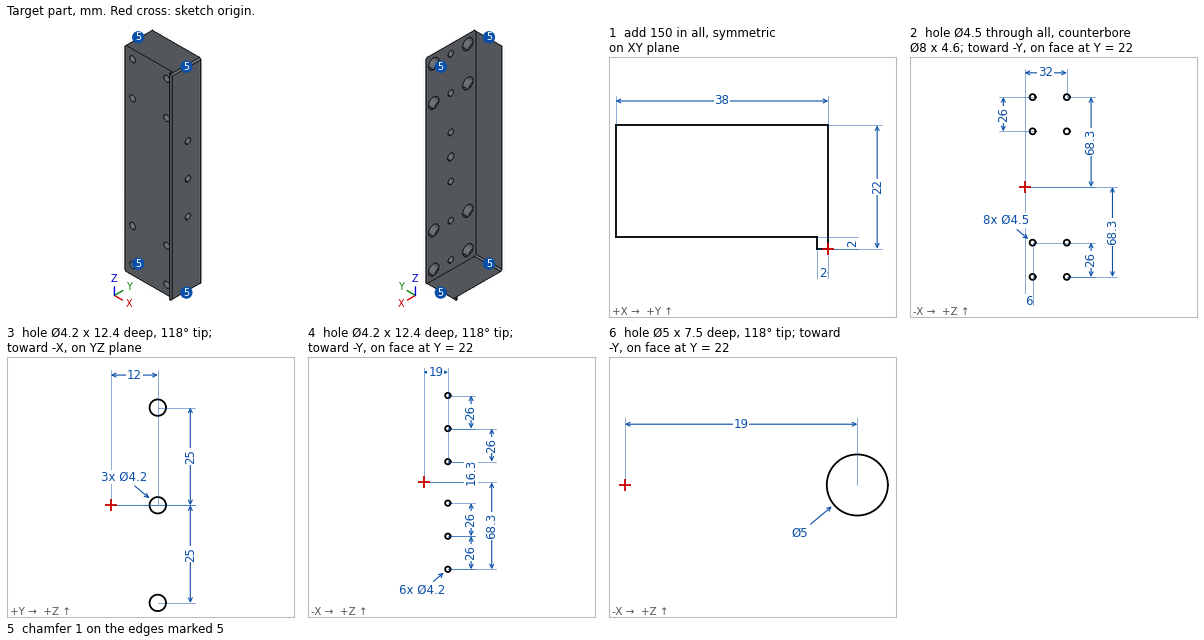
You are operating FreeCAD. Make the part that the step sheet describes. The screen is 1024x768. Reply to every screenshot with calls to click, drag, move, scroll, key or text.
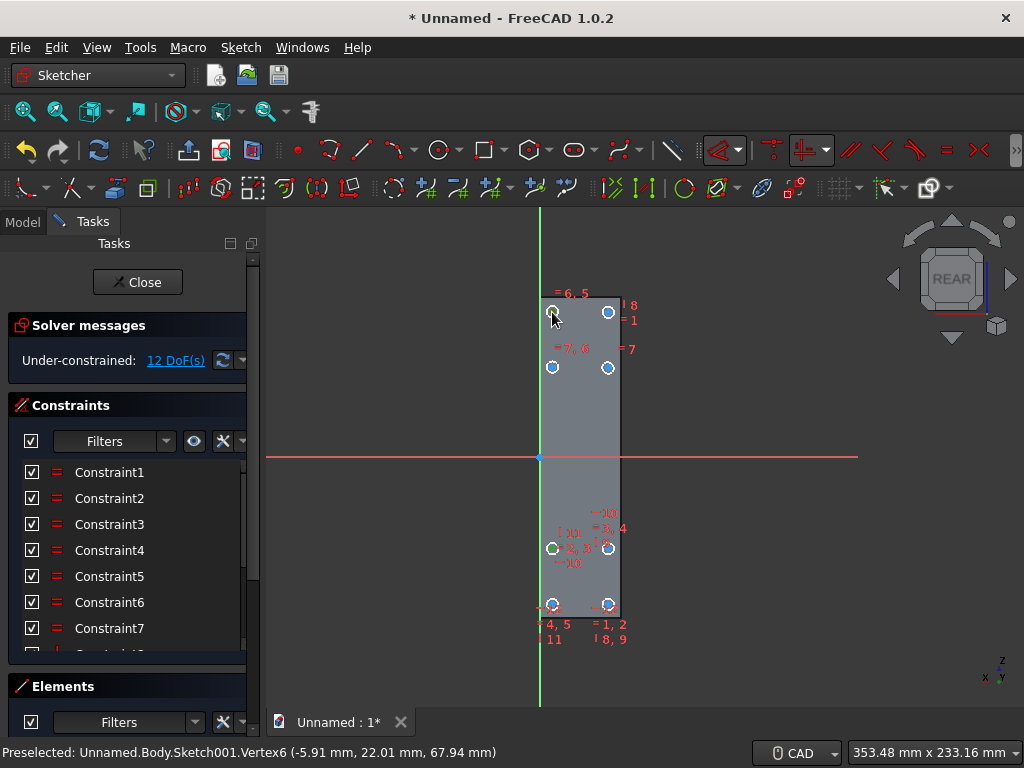
key(v)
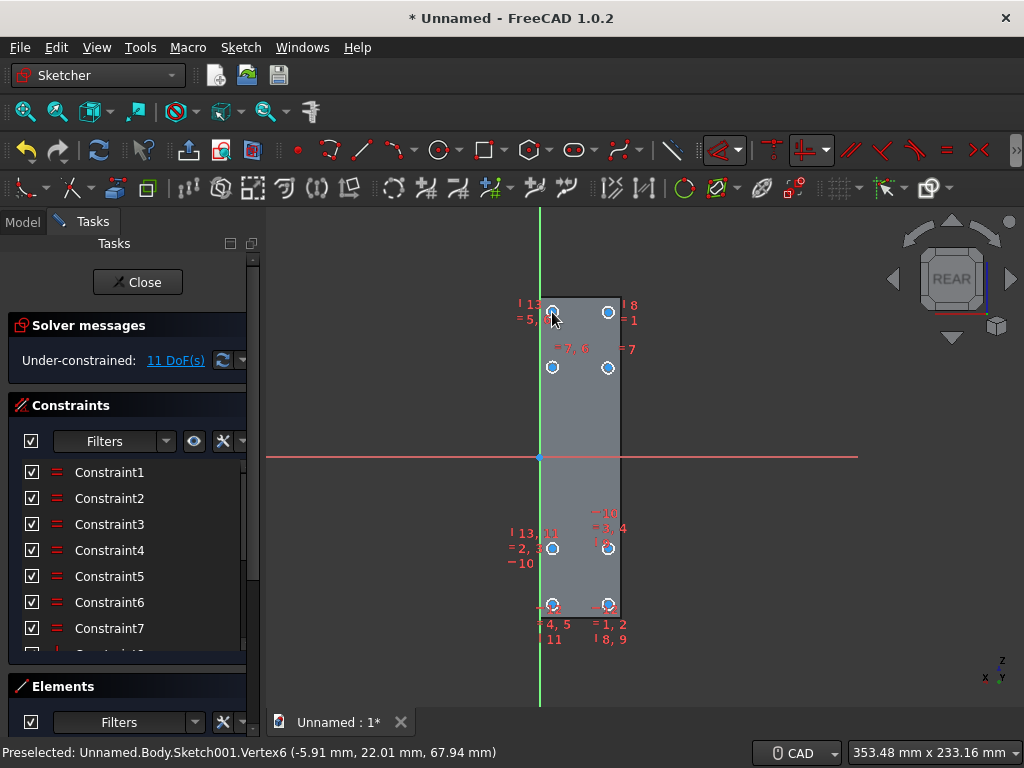
click(608, 312)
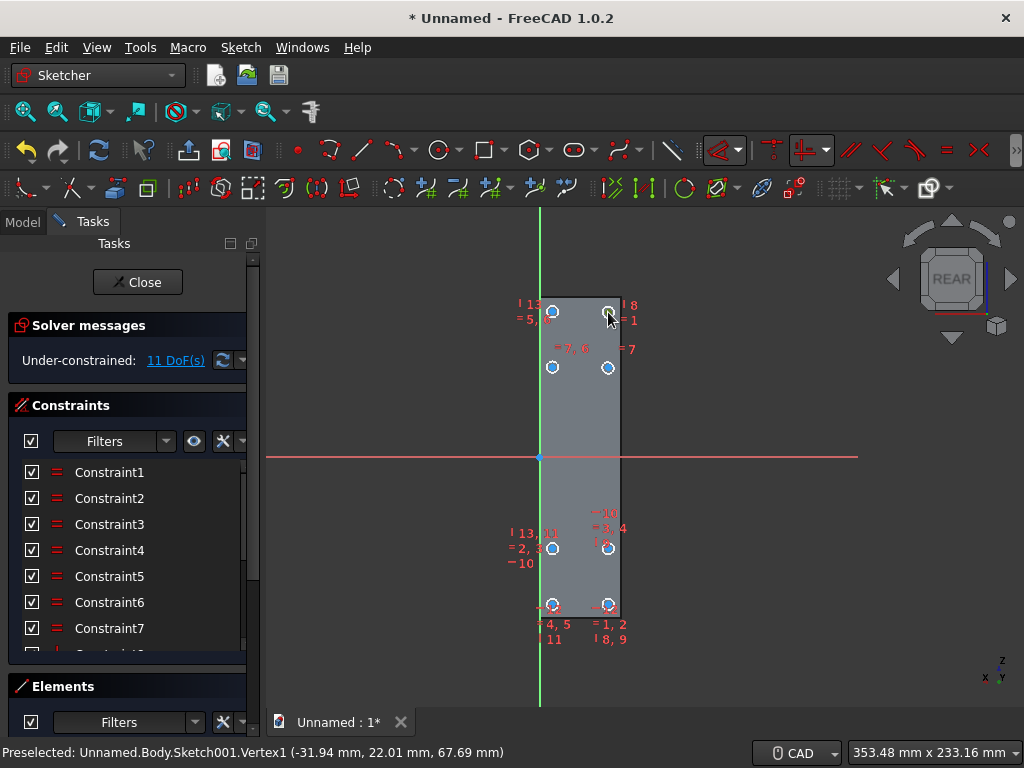
click(553, 312)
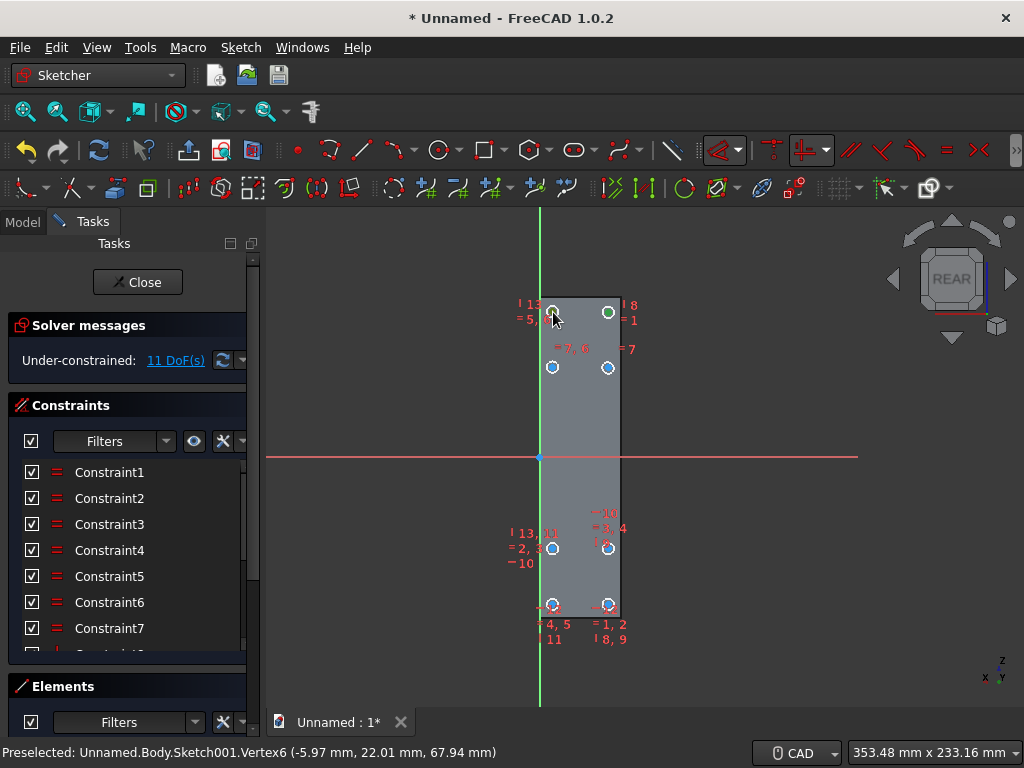
key(h)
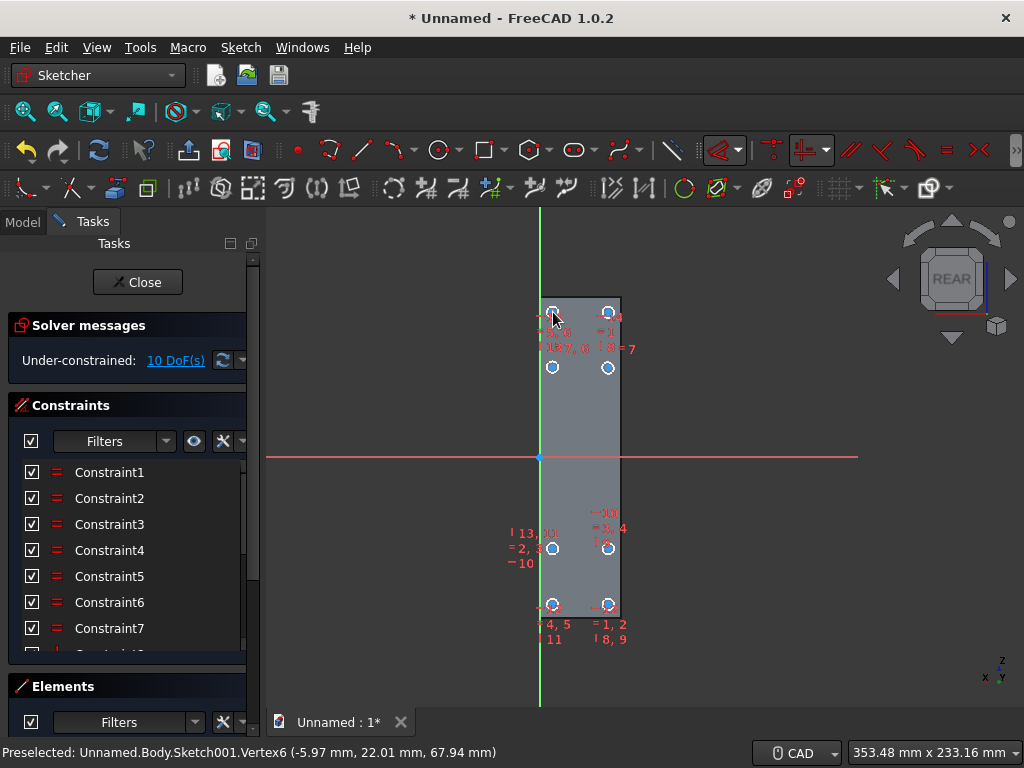
scroll(553, 312, up, 4)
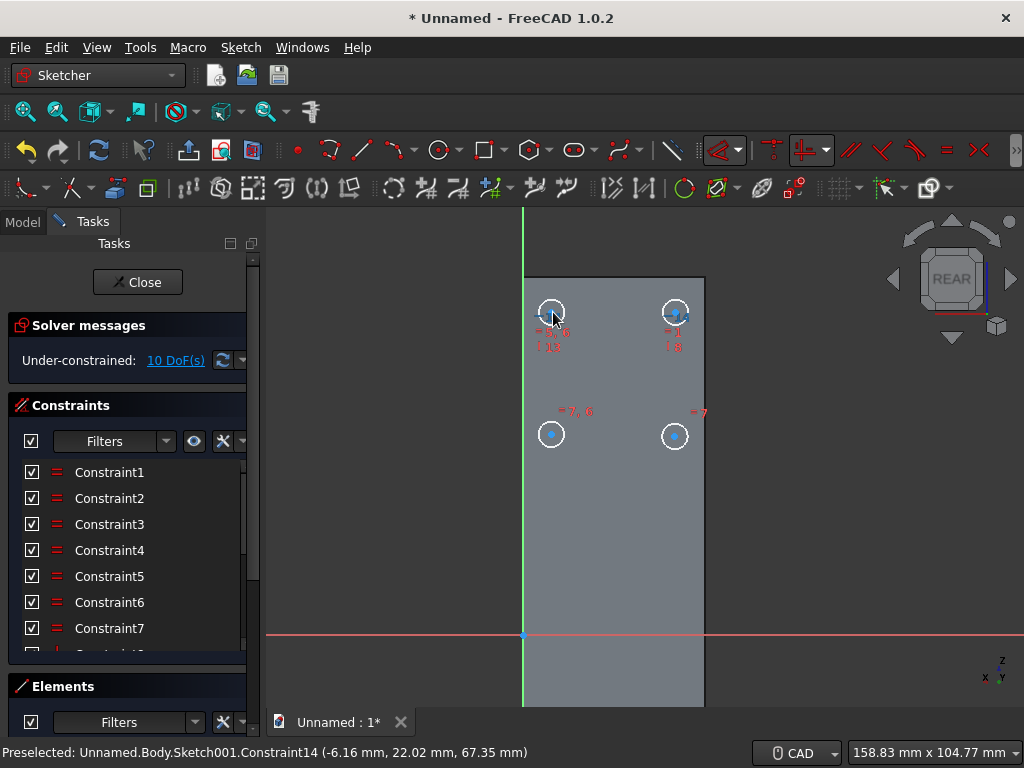
scroll(552, 312, up, 4)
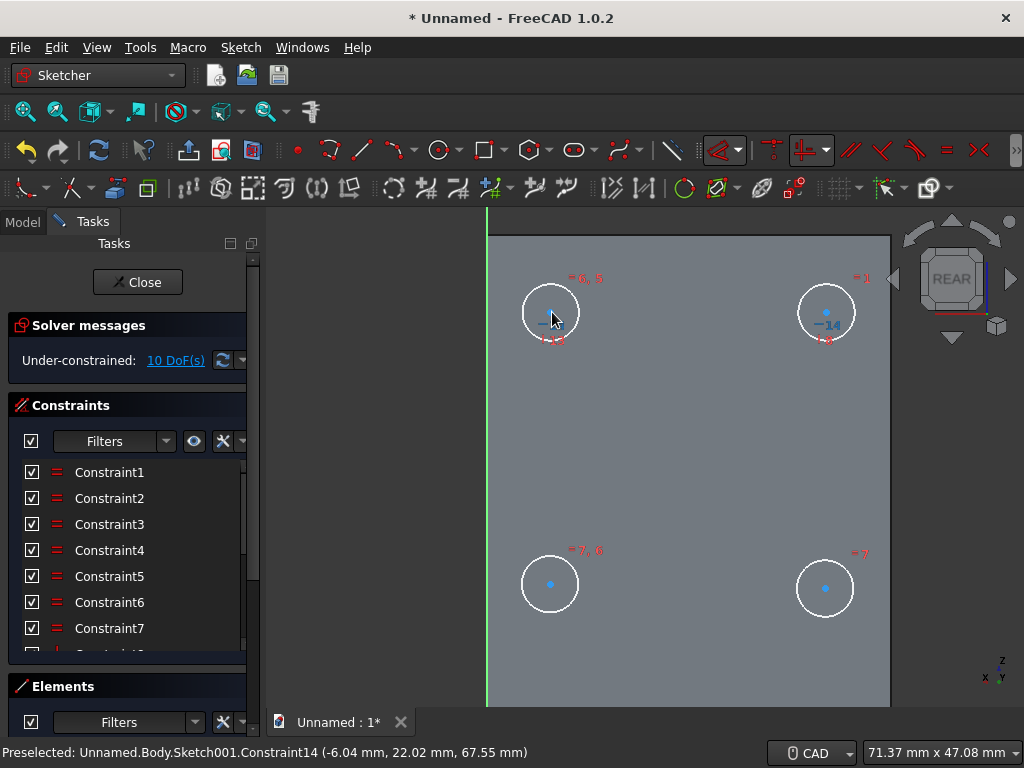
click(551, 312)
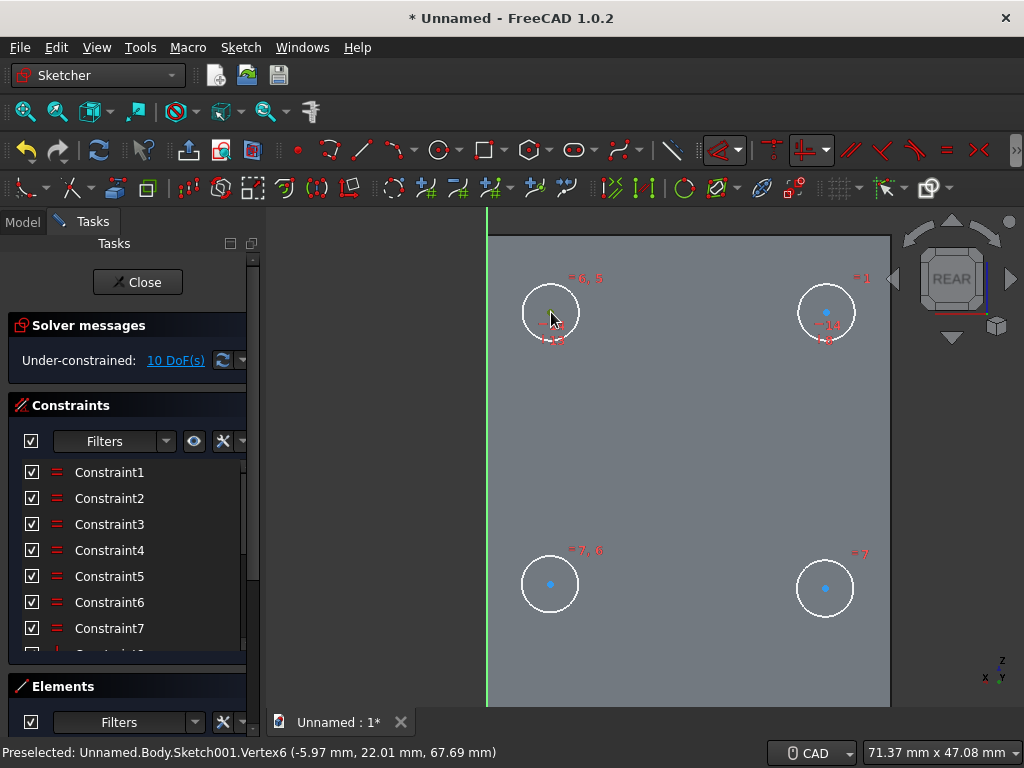
scroll(553, 312, down, 8)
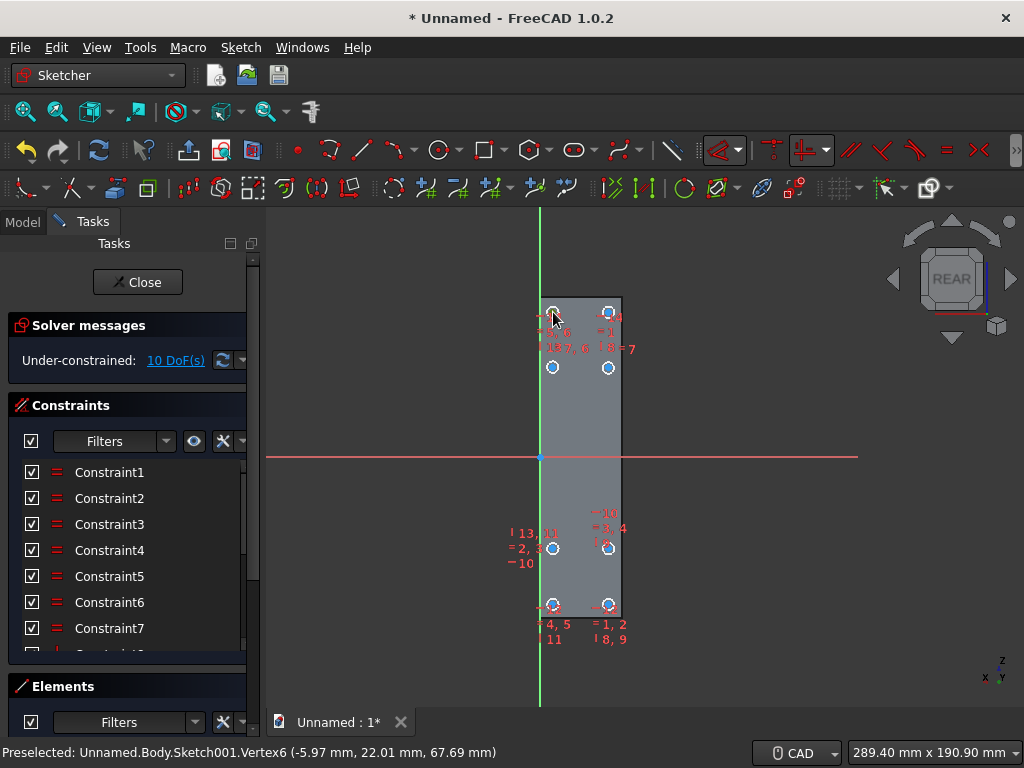
click(553, 367)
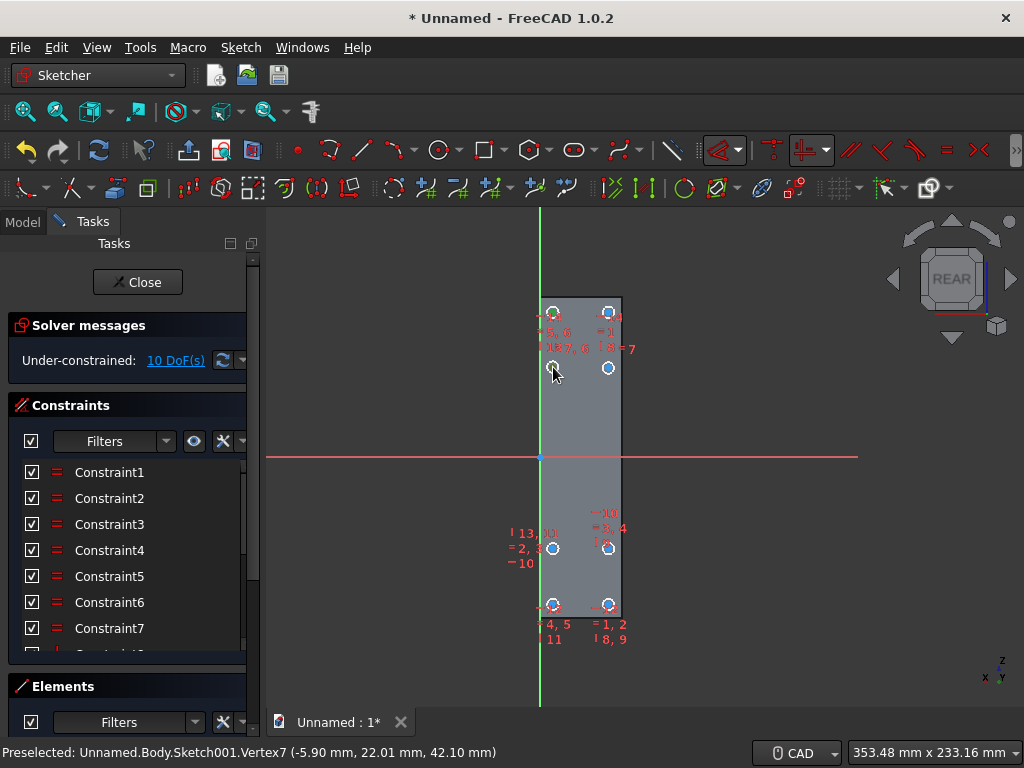
key(v)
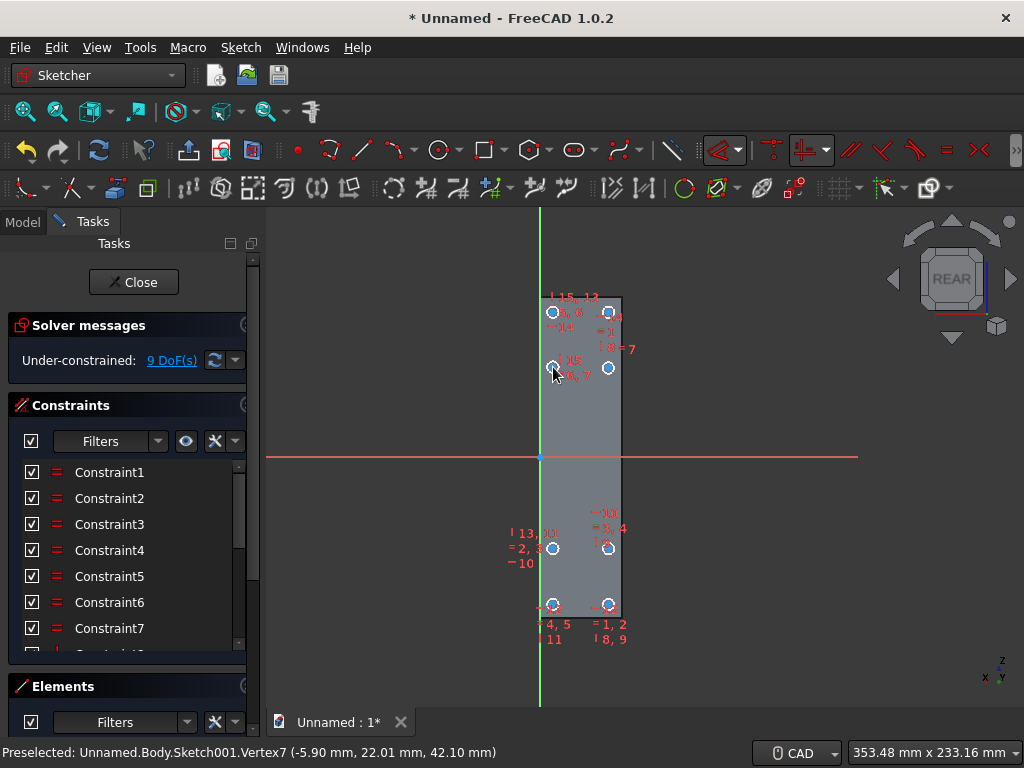
click(609, 312)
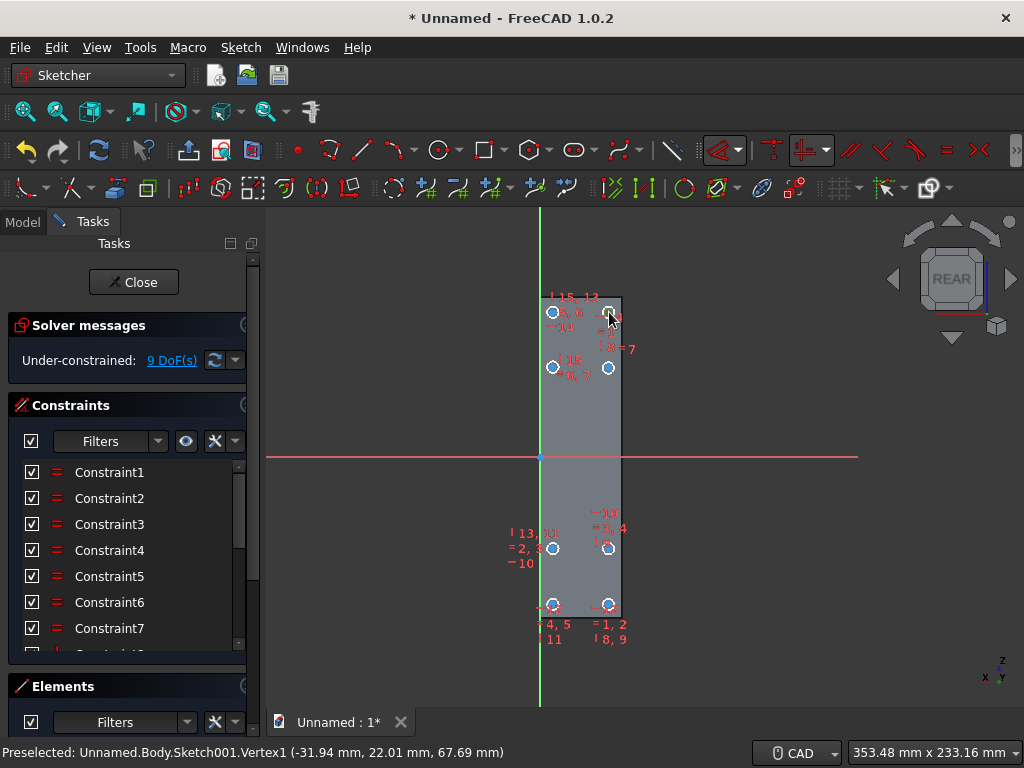
click(608, 368)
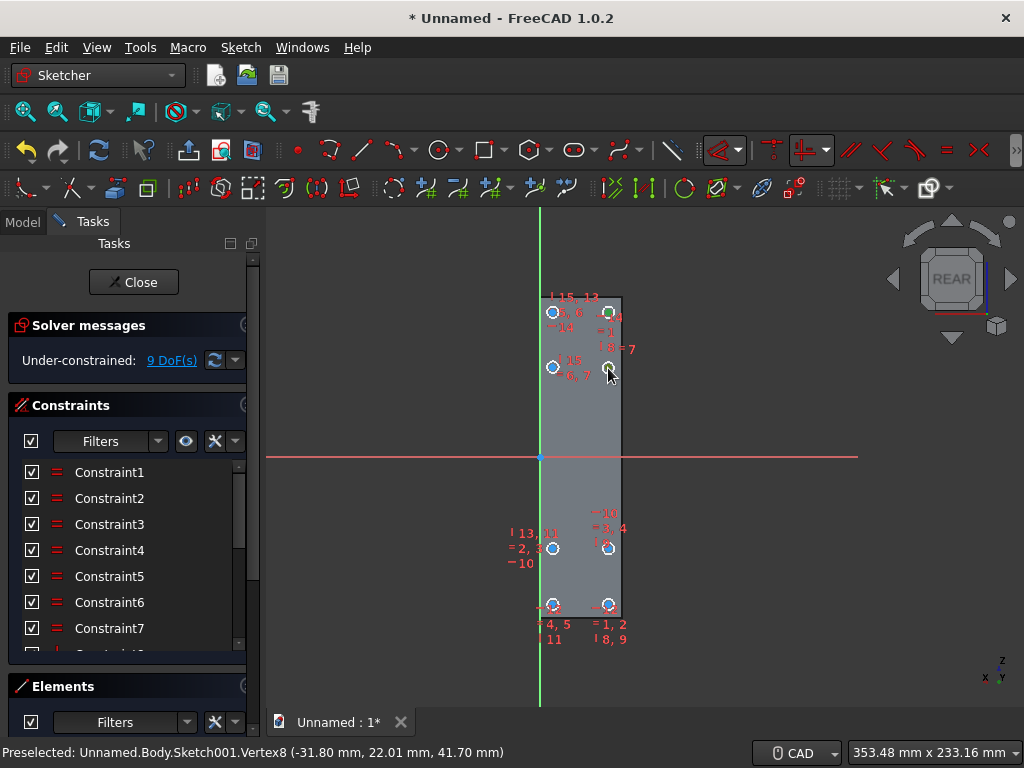
key(v)